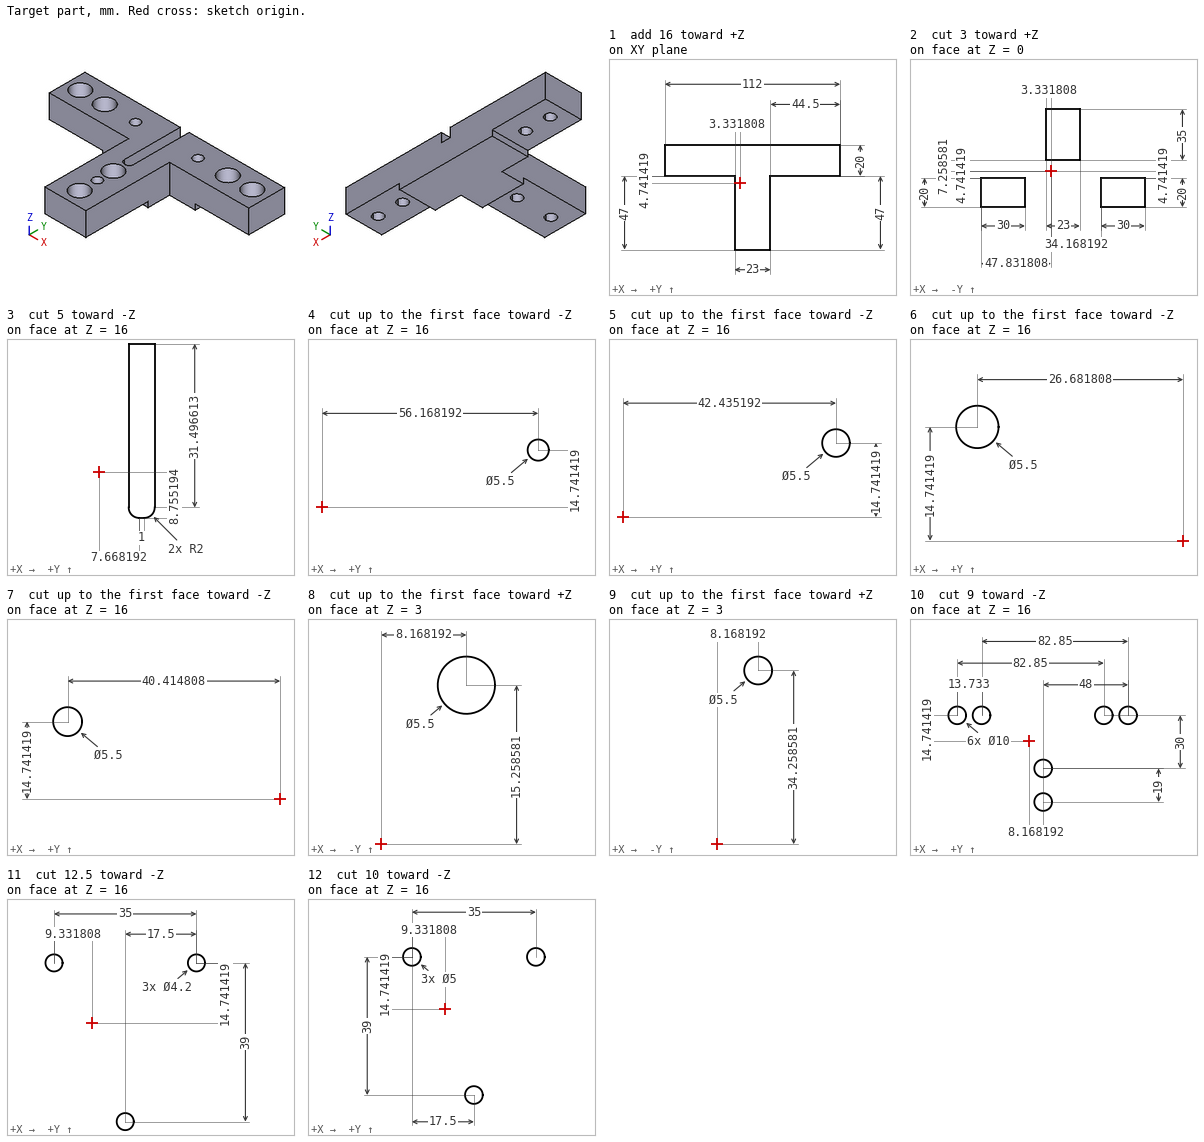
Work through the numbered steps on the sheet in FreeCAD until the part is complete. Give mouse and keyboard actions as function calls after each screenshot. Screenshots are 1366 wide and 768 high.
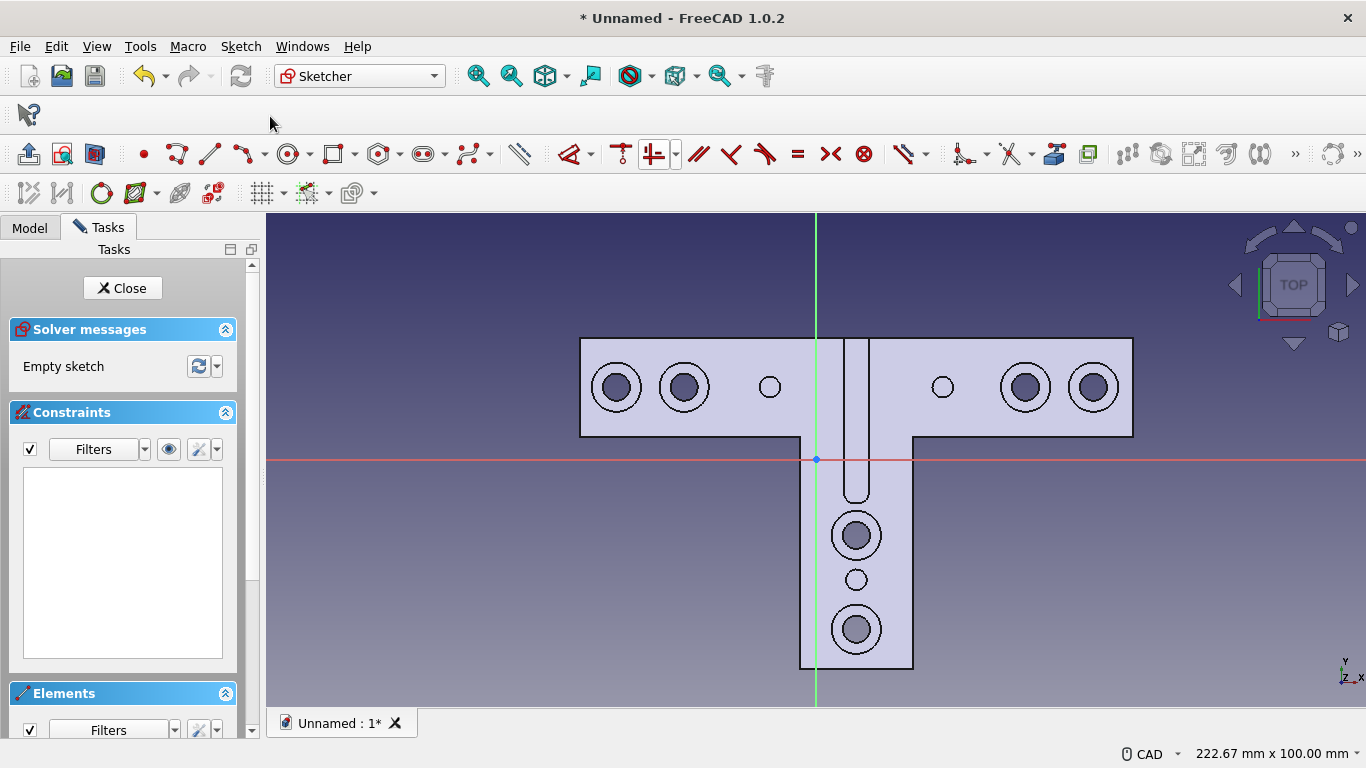
scroll(1078, 531, up, 2)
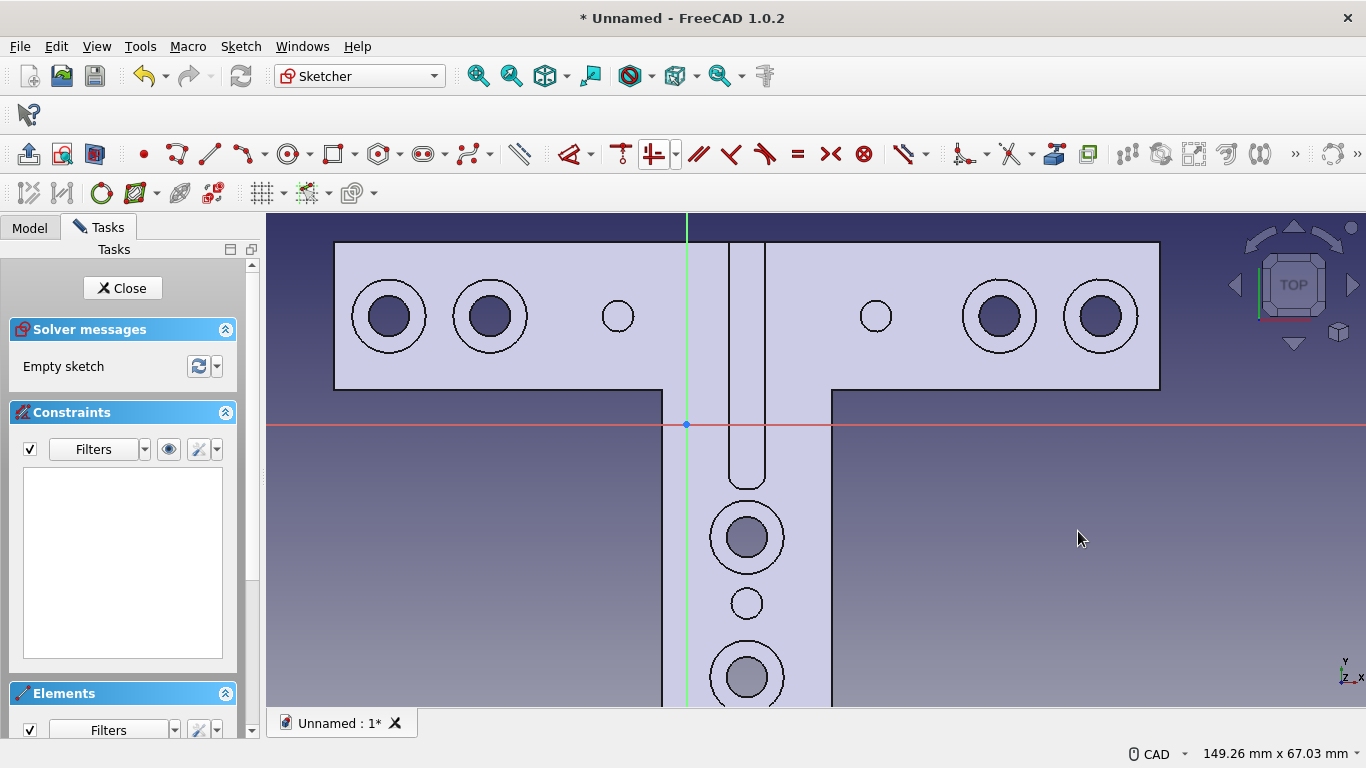
click(288, 154)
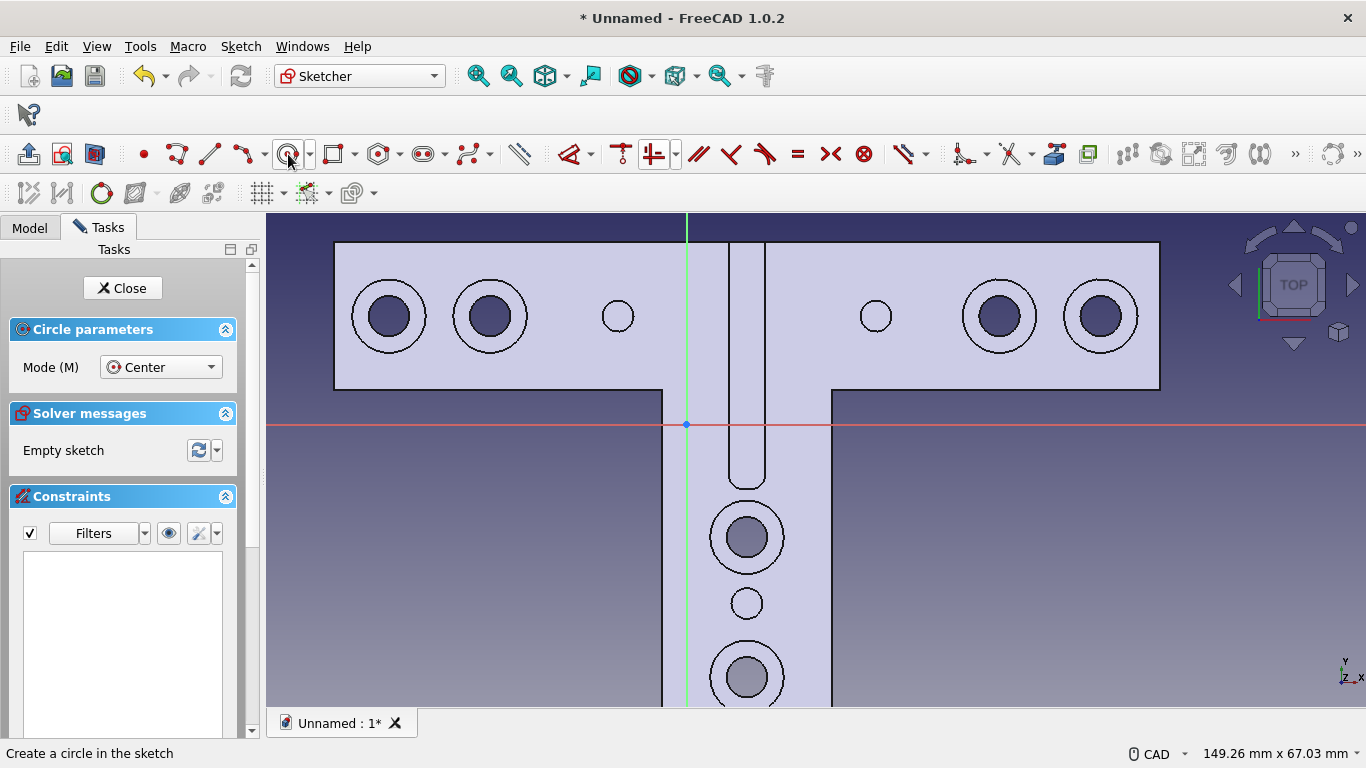
scroll(618, 316, up, 2)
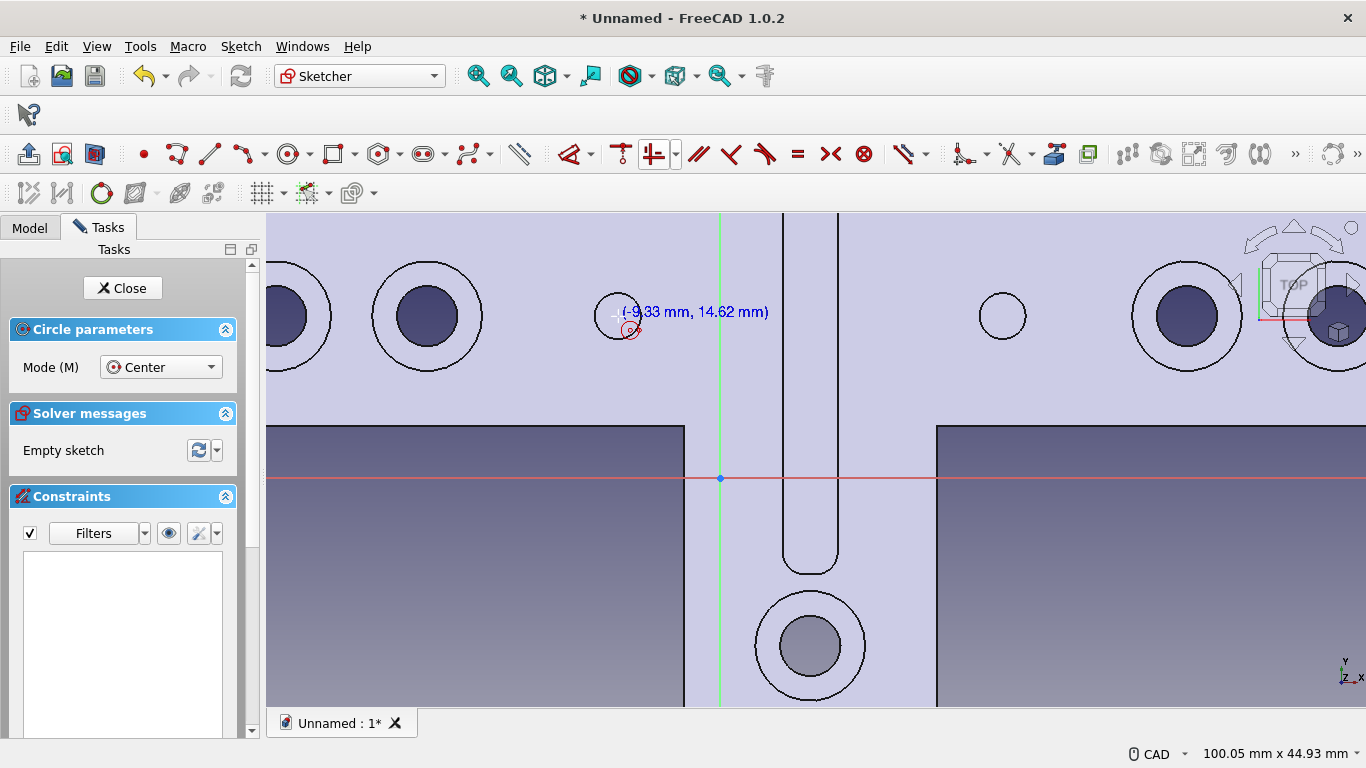
click(618, 316)
move(637, 297)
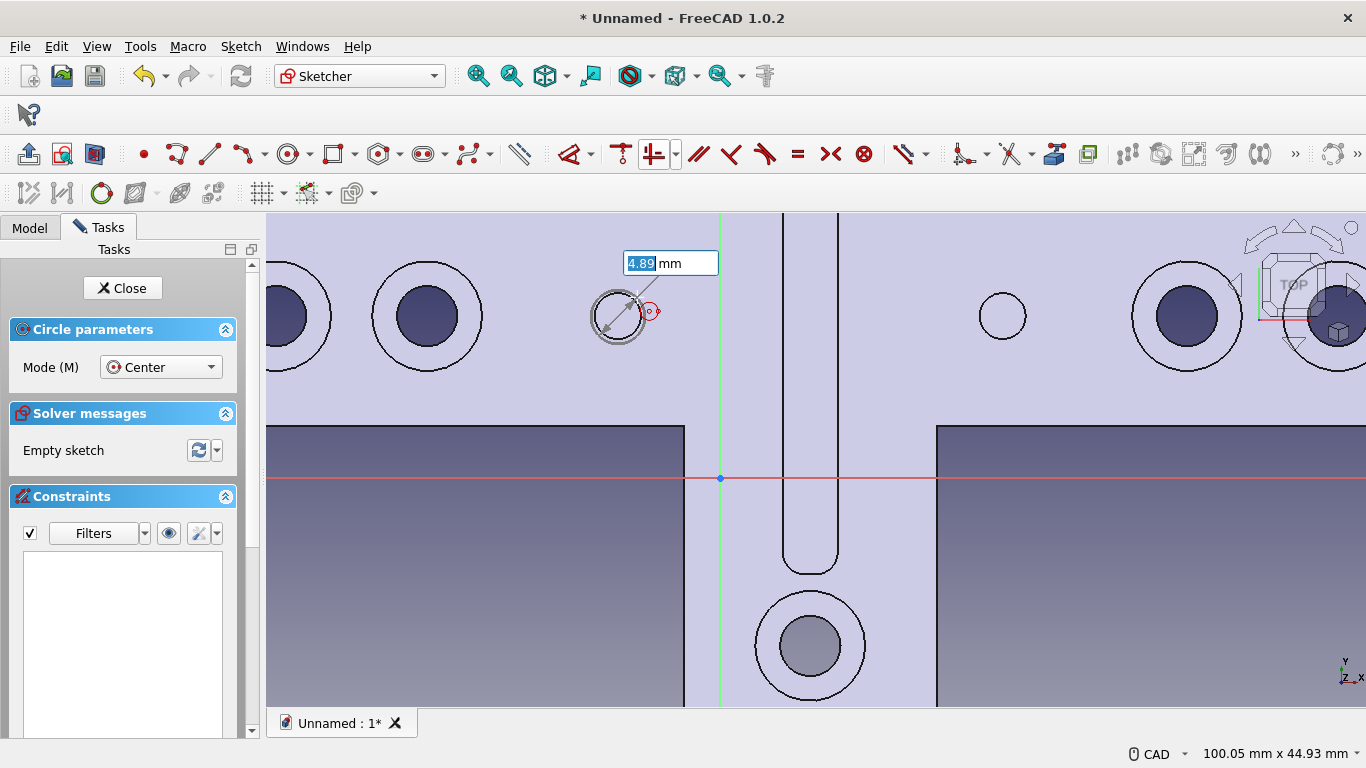
text(5)
key(Return)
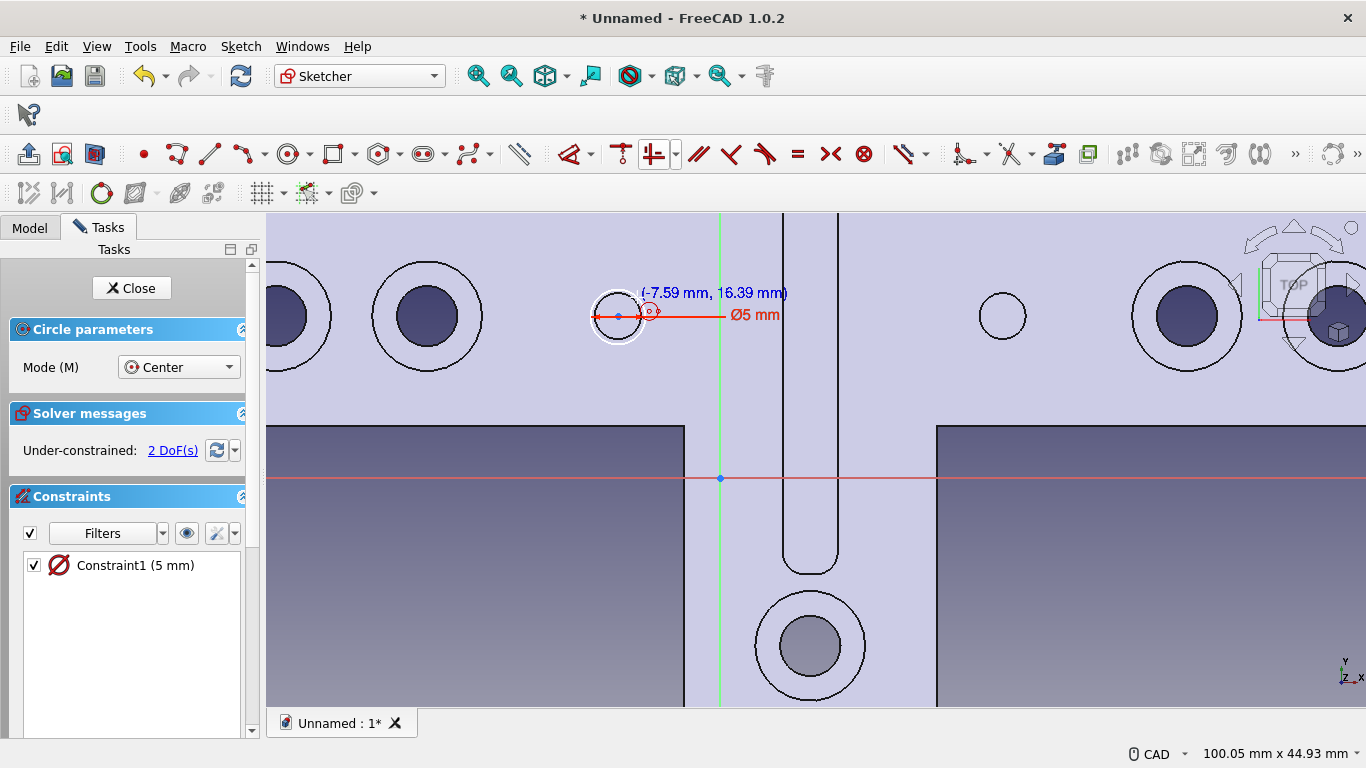
click(1003, 316)
move(1022, 297)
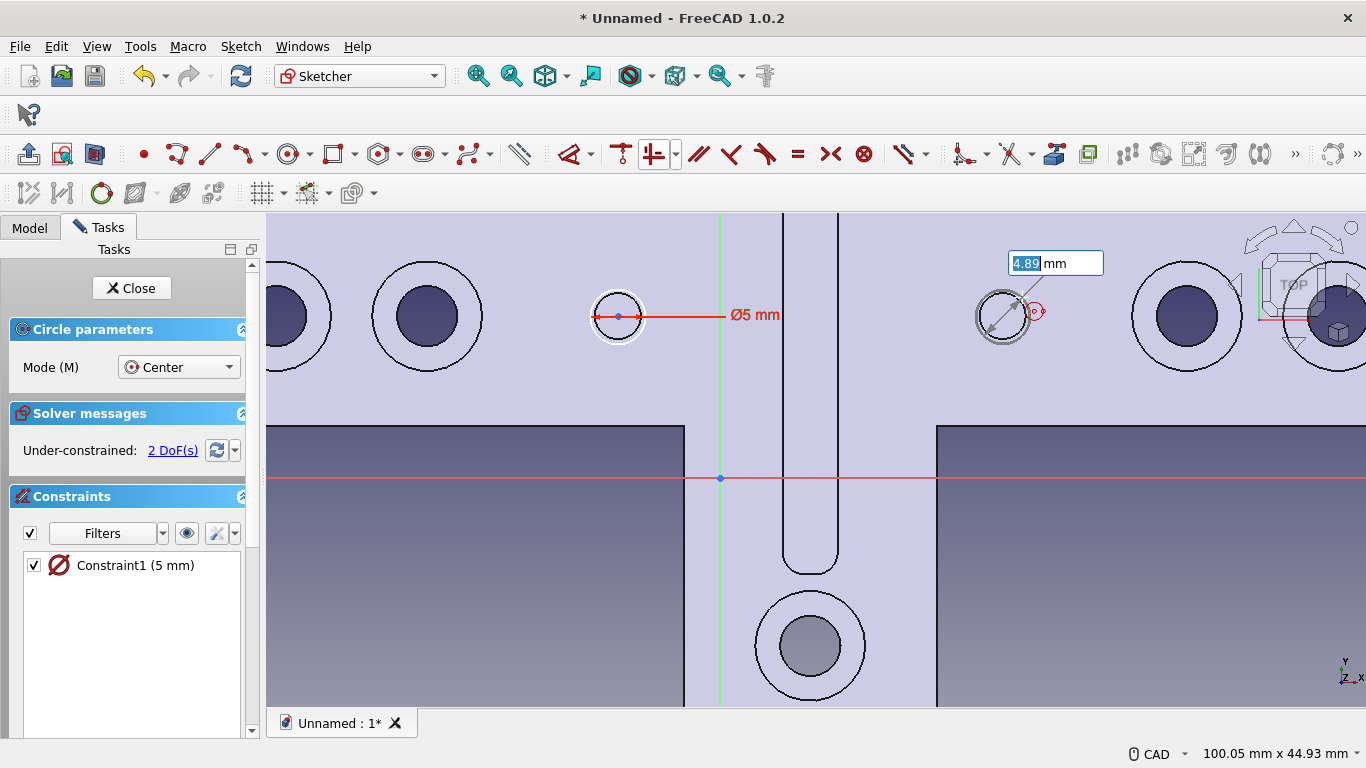
text(5)
key(Return)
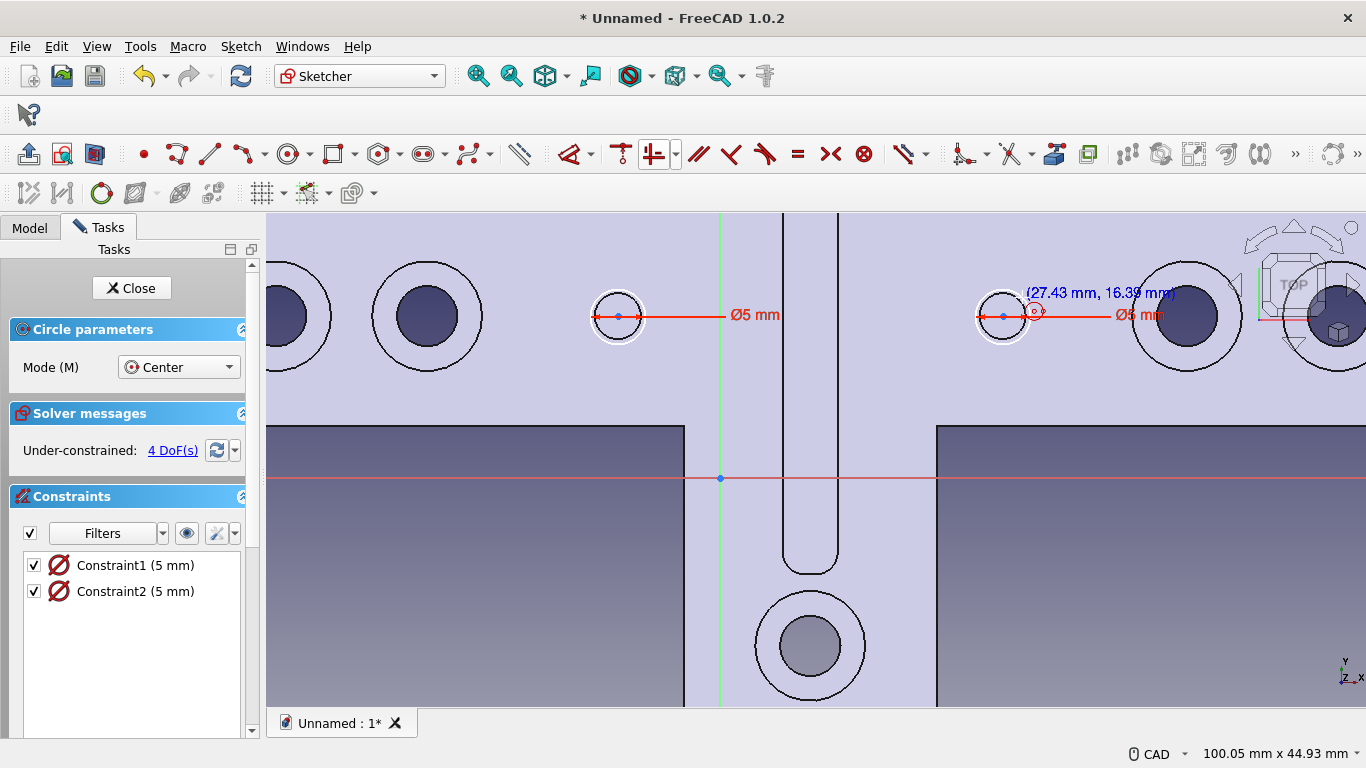
scroll(620, 317, down, 2)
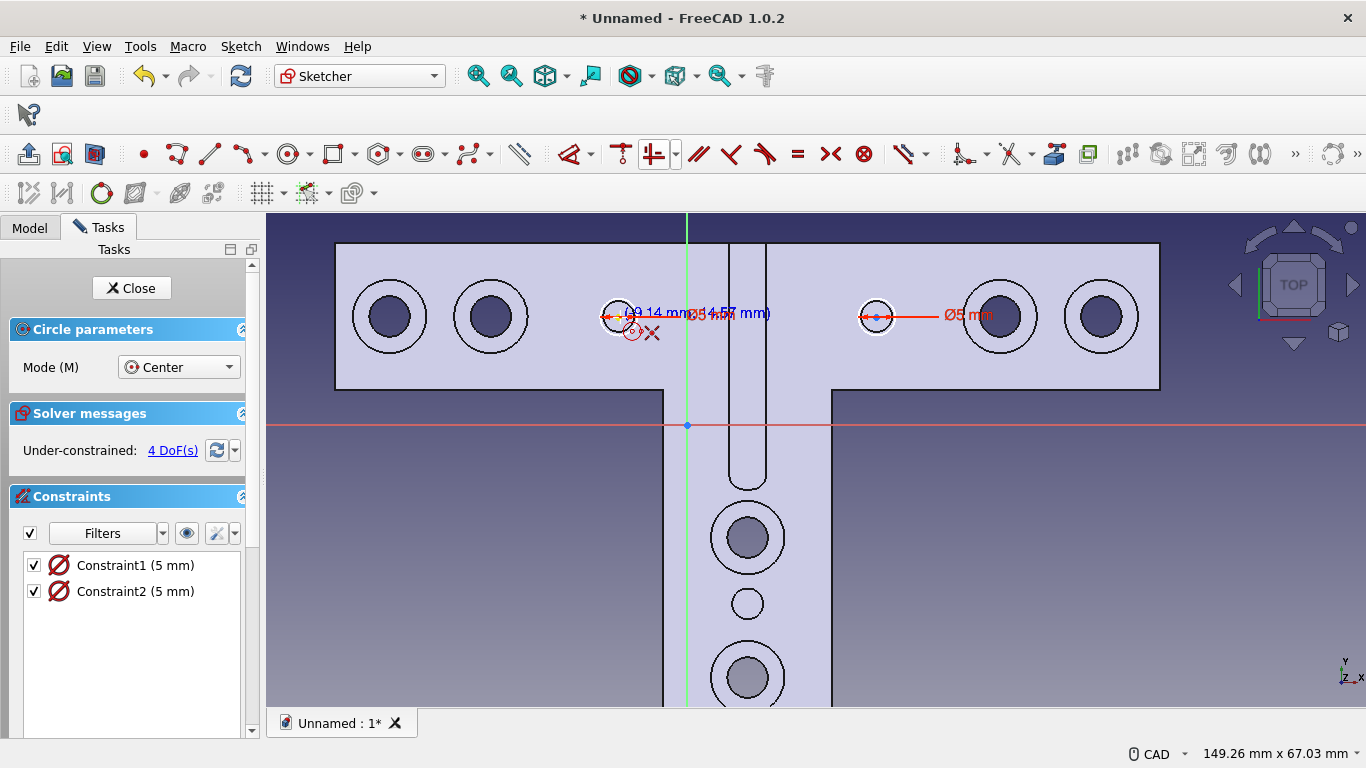
scroll(748, 604, up, 2)